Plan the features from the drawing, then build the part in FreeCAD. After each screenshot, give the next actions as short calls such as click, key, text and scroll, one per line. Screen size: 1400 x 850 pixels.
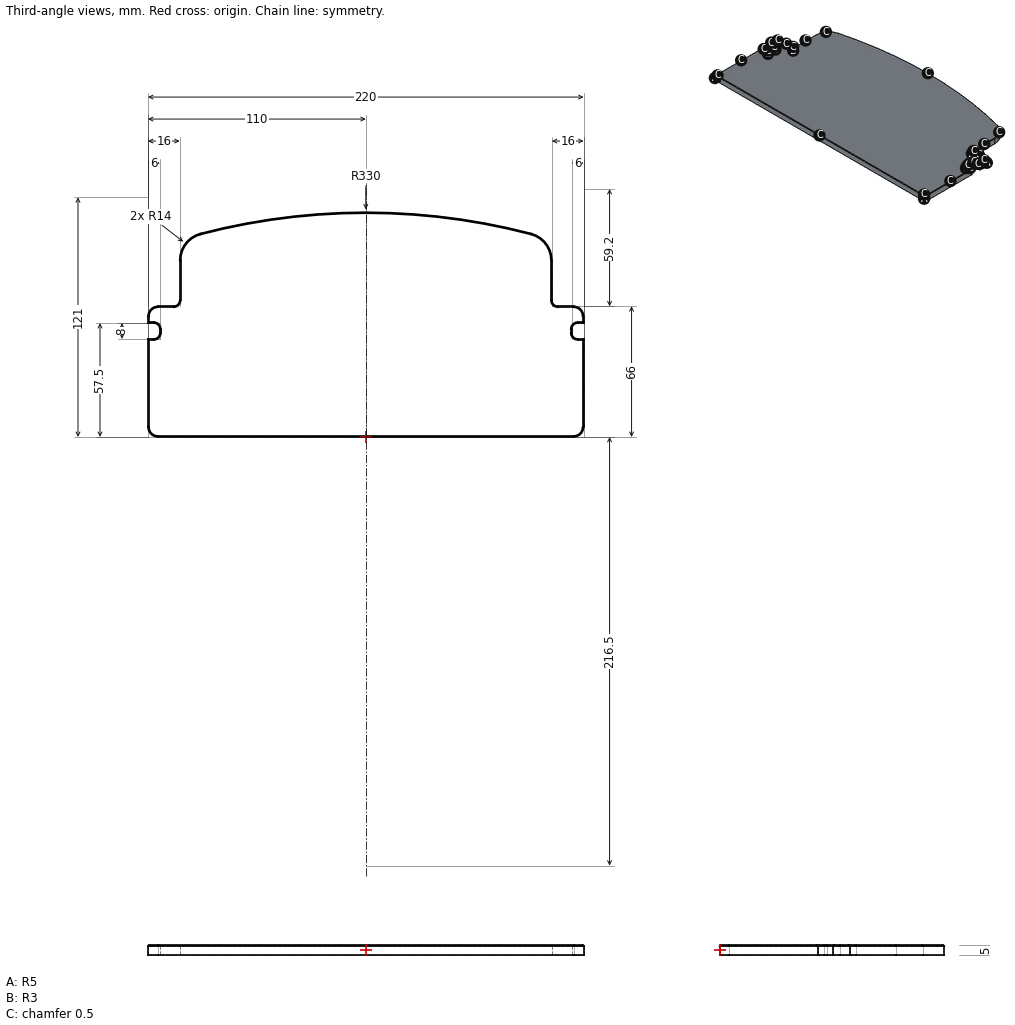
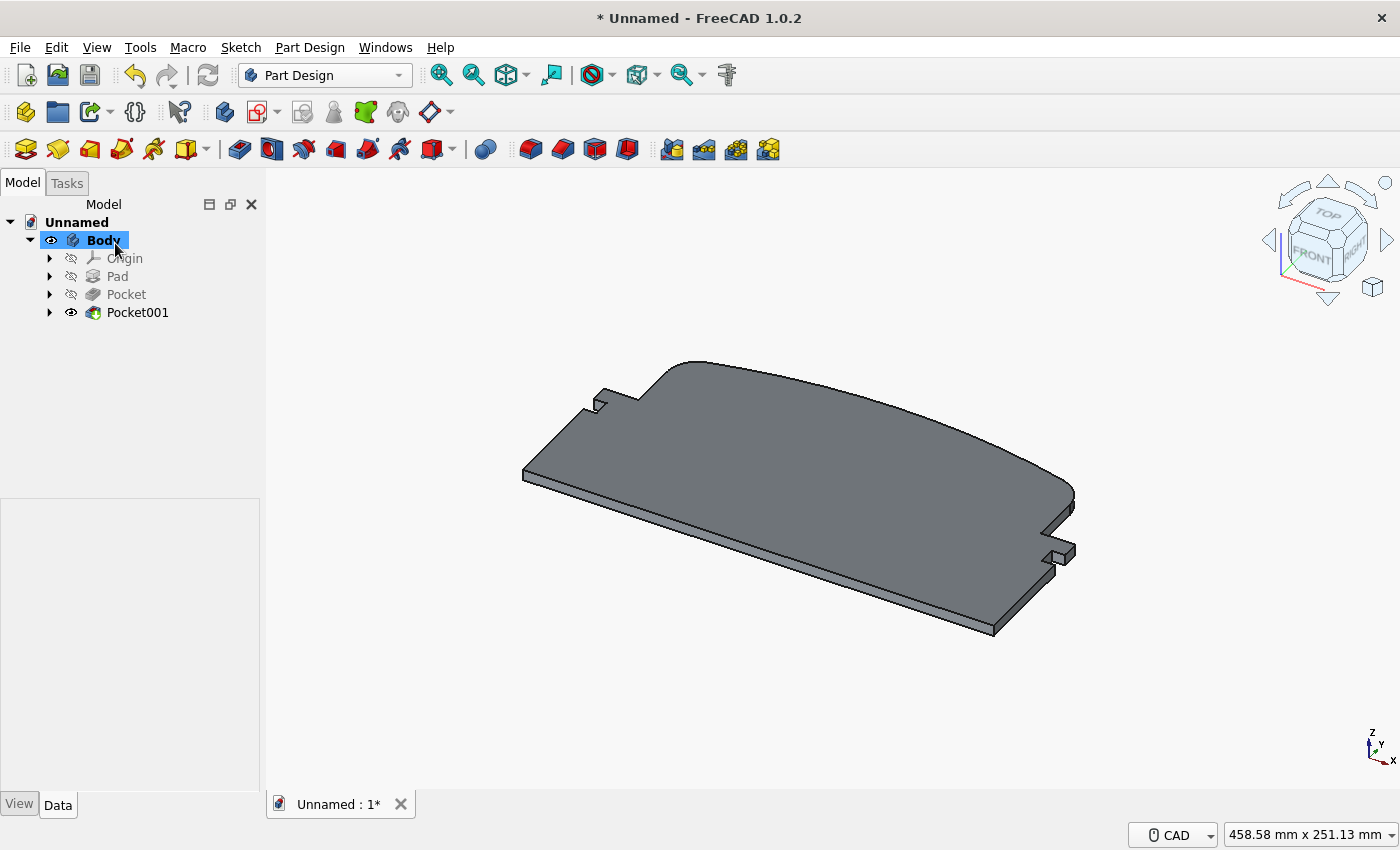
click(994, 631)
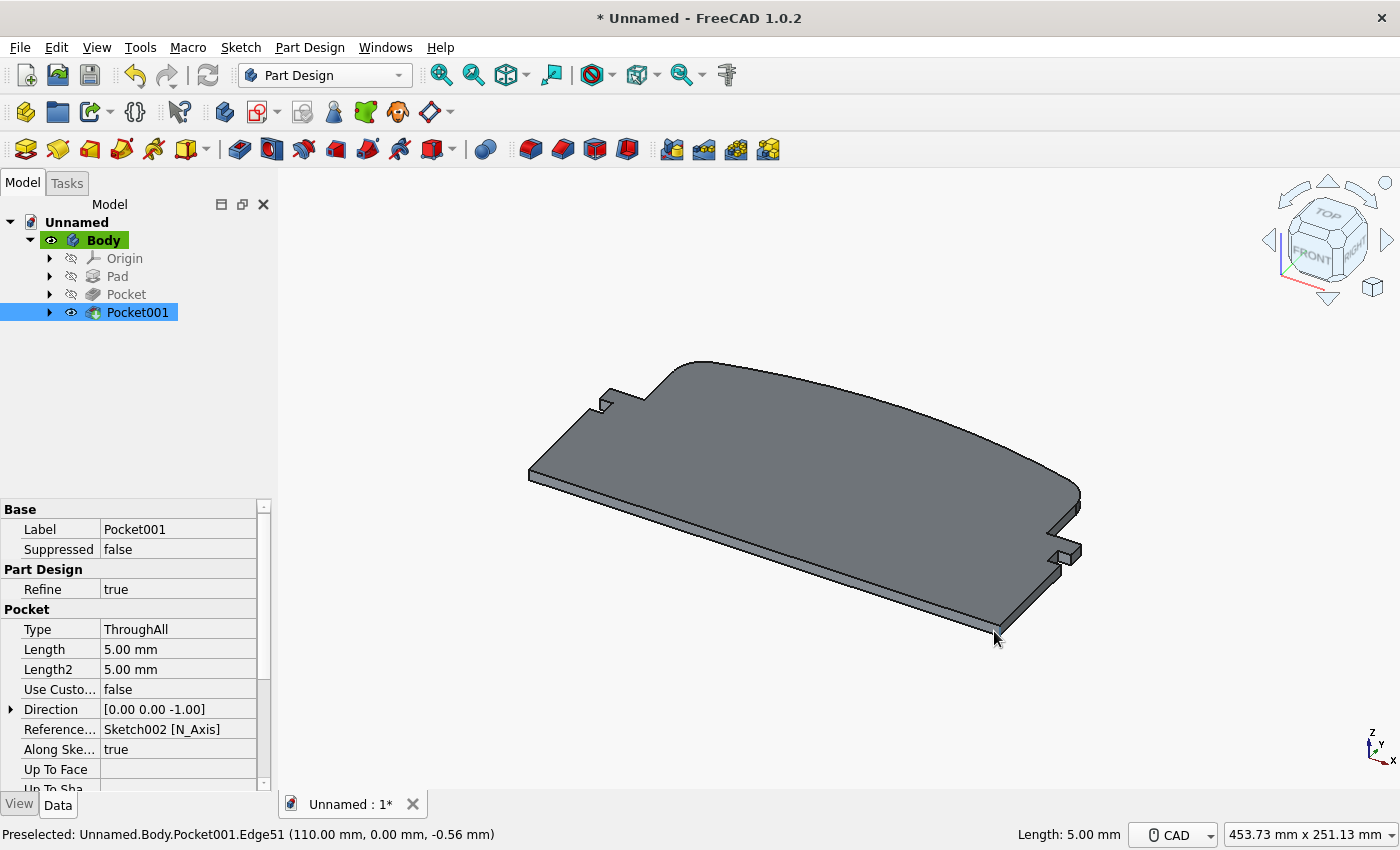
scroll(610, 393, up, 6)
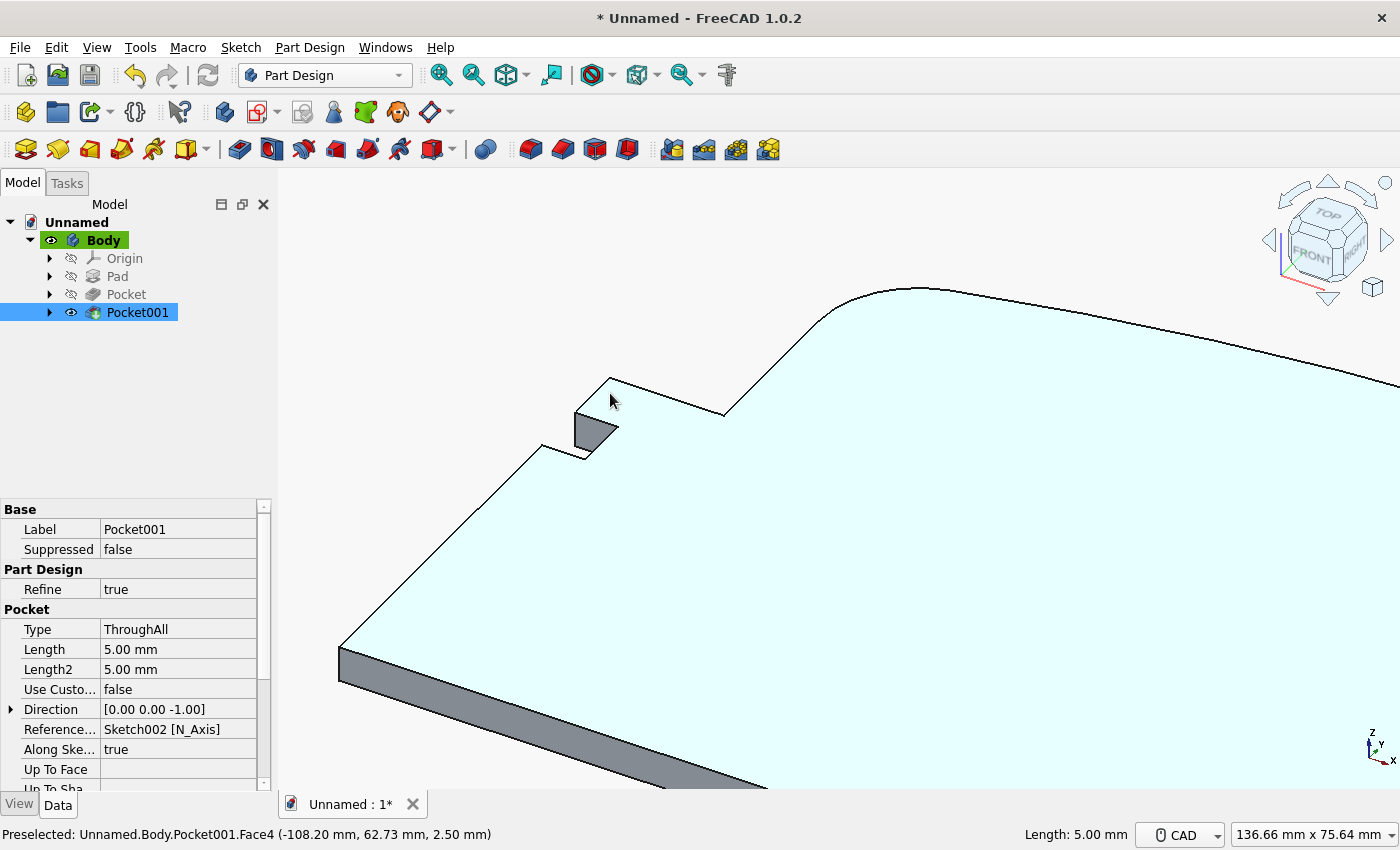
key(v)
key(f)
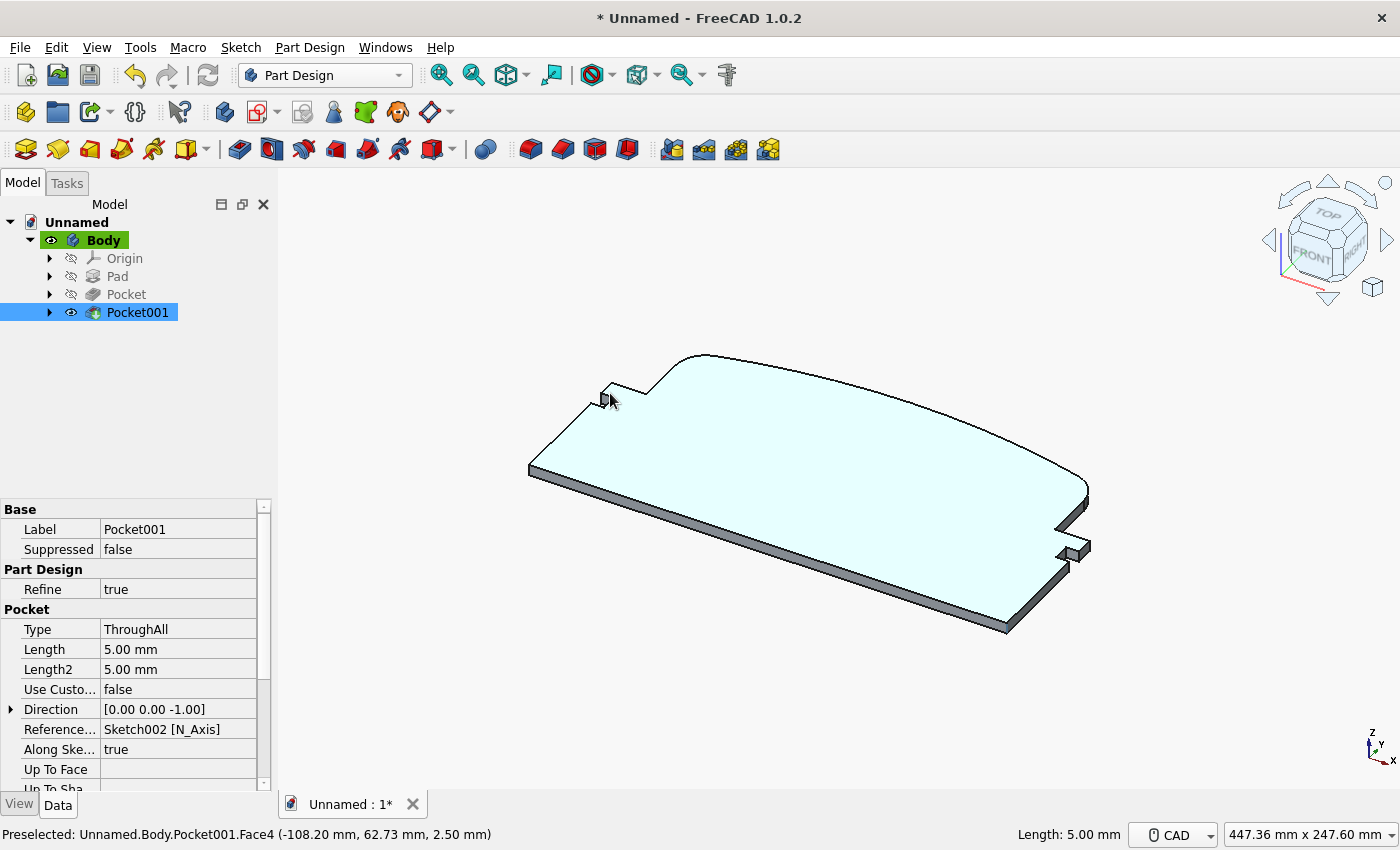
key(0)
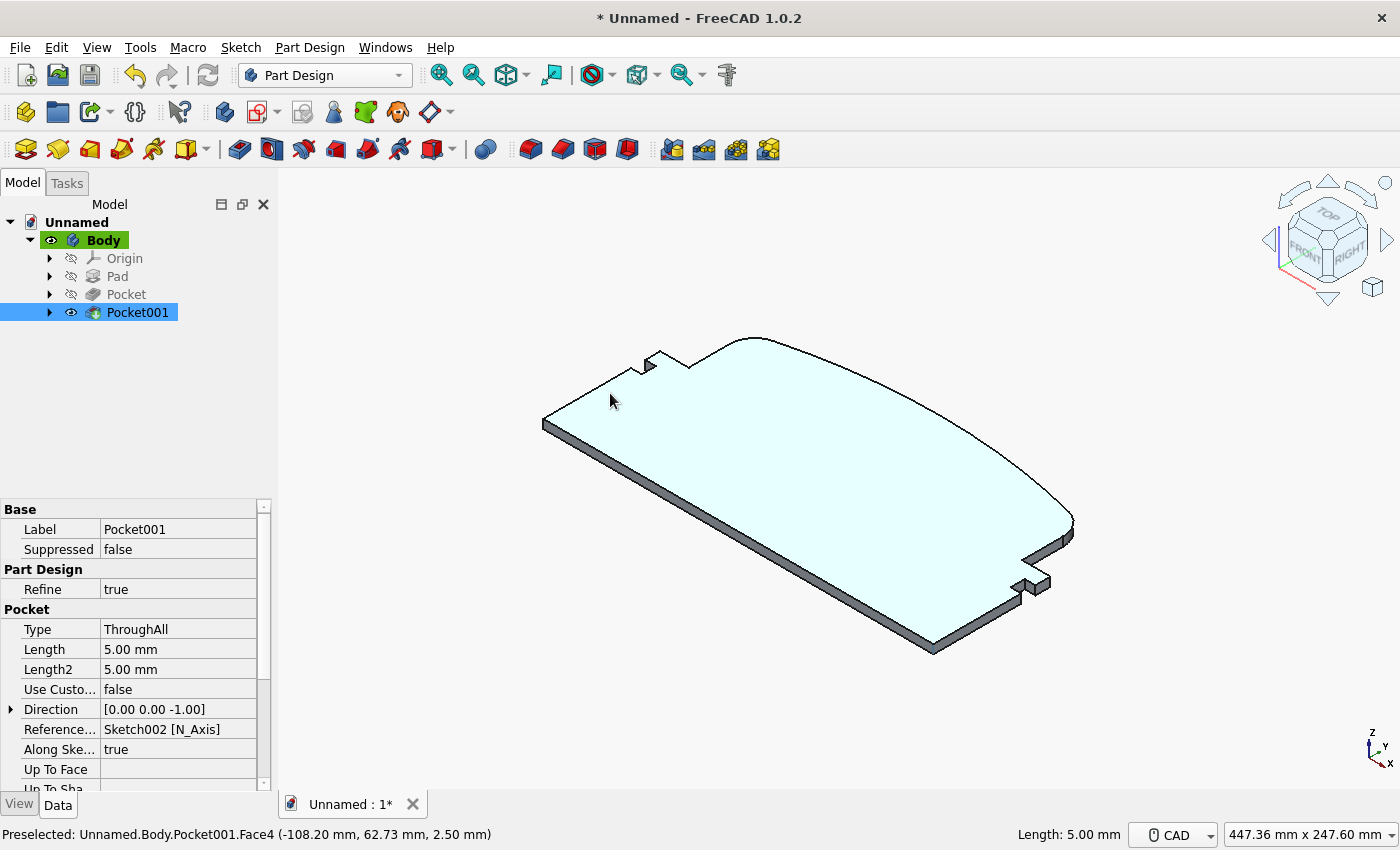
scroll(660, 355, up, 6)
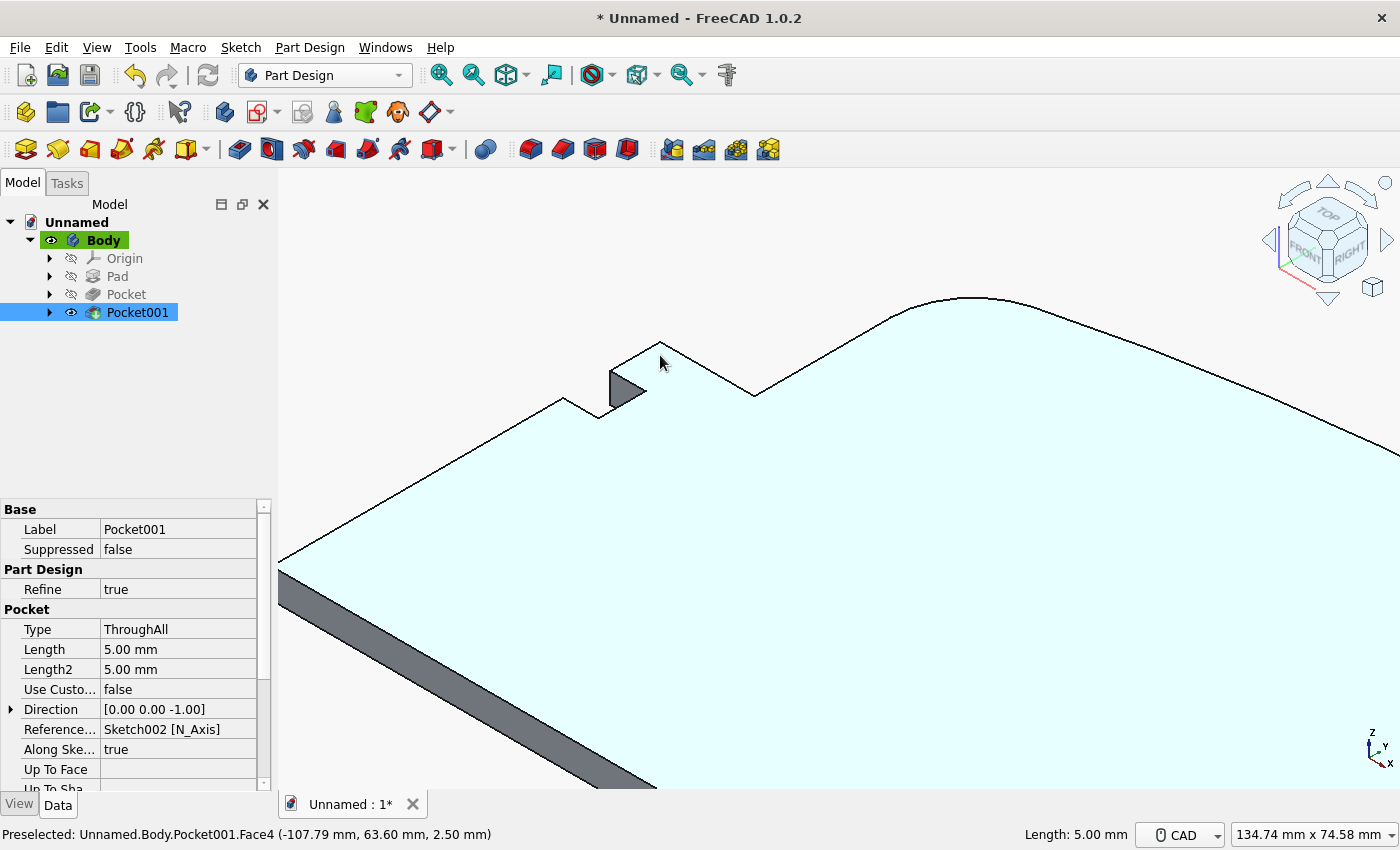
click(442, 76)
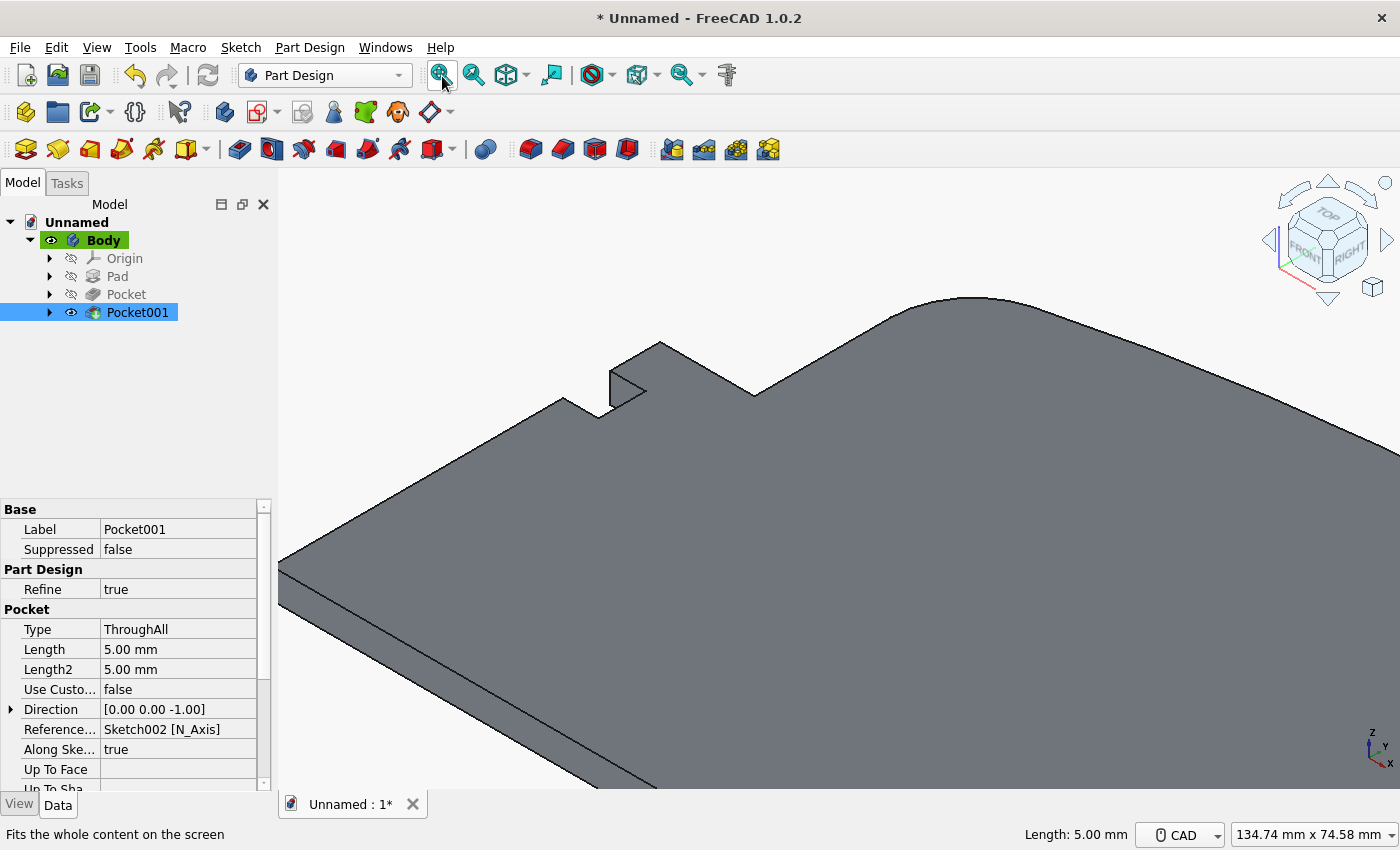
key(2)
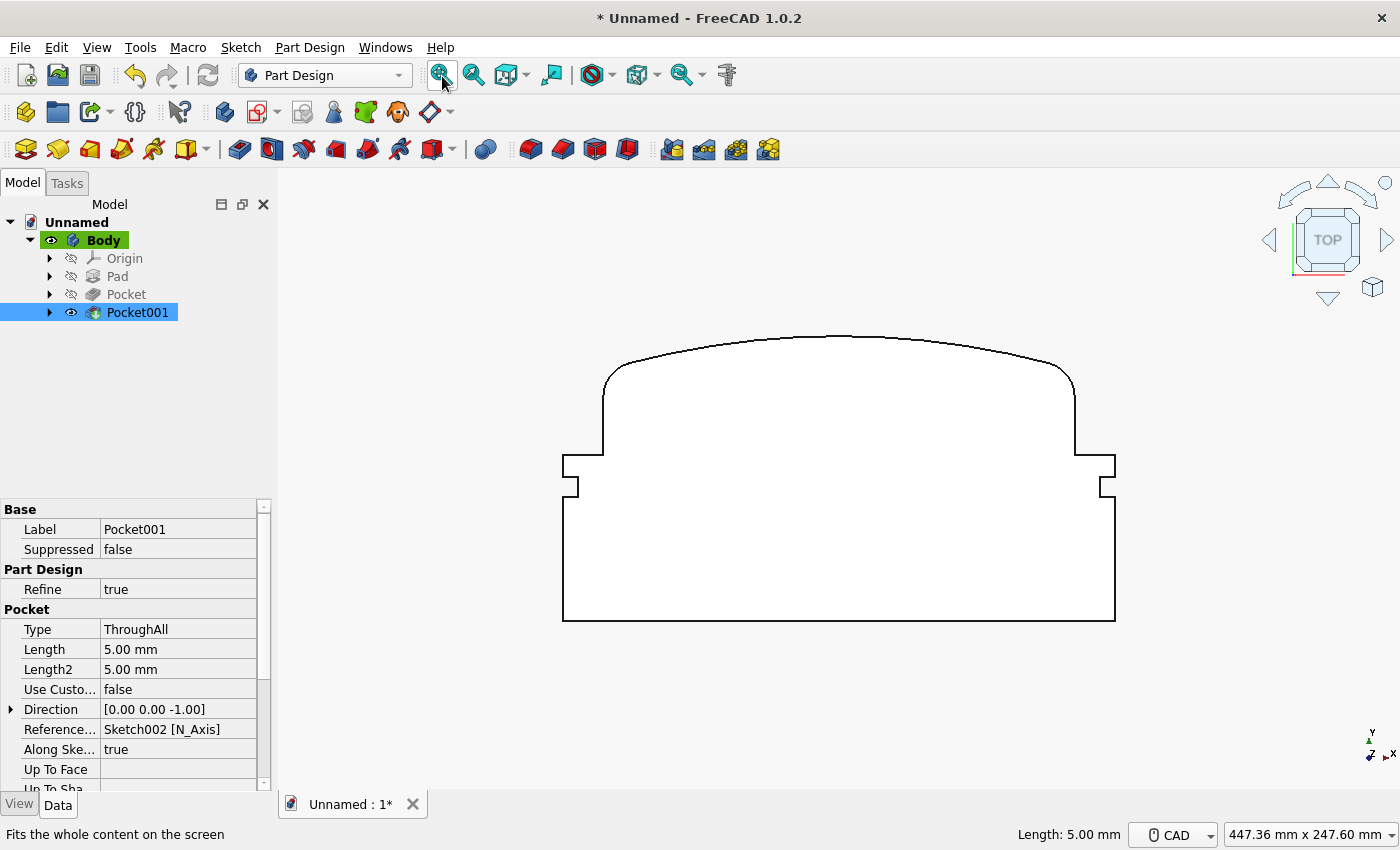
scroll(563, 454, up, 6)